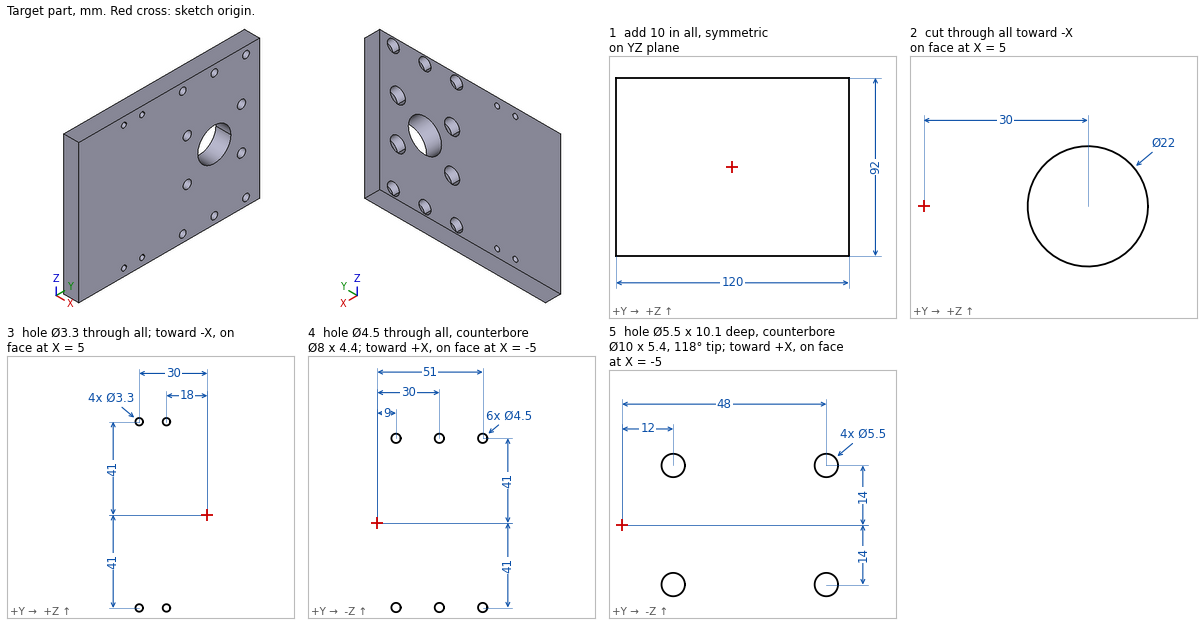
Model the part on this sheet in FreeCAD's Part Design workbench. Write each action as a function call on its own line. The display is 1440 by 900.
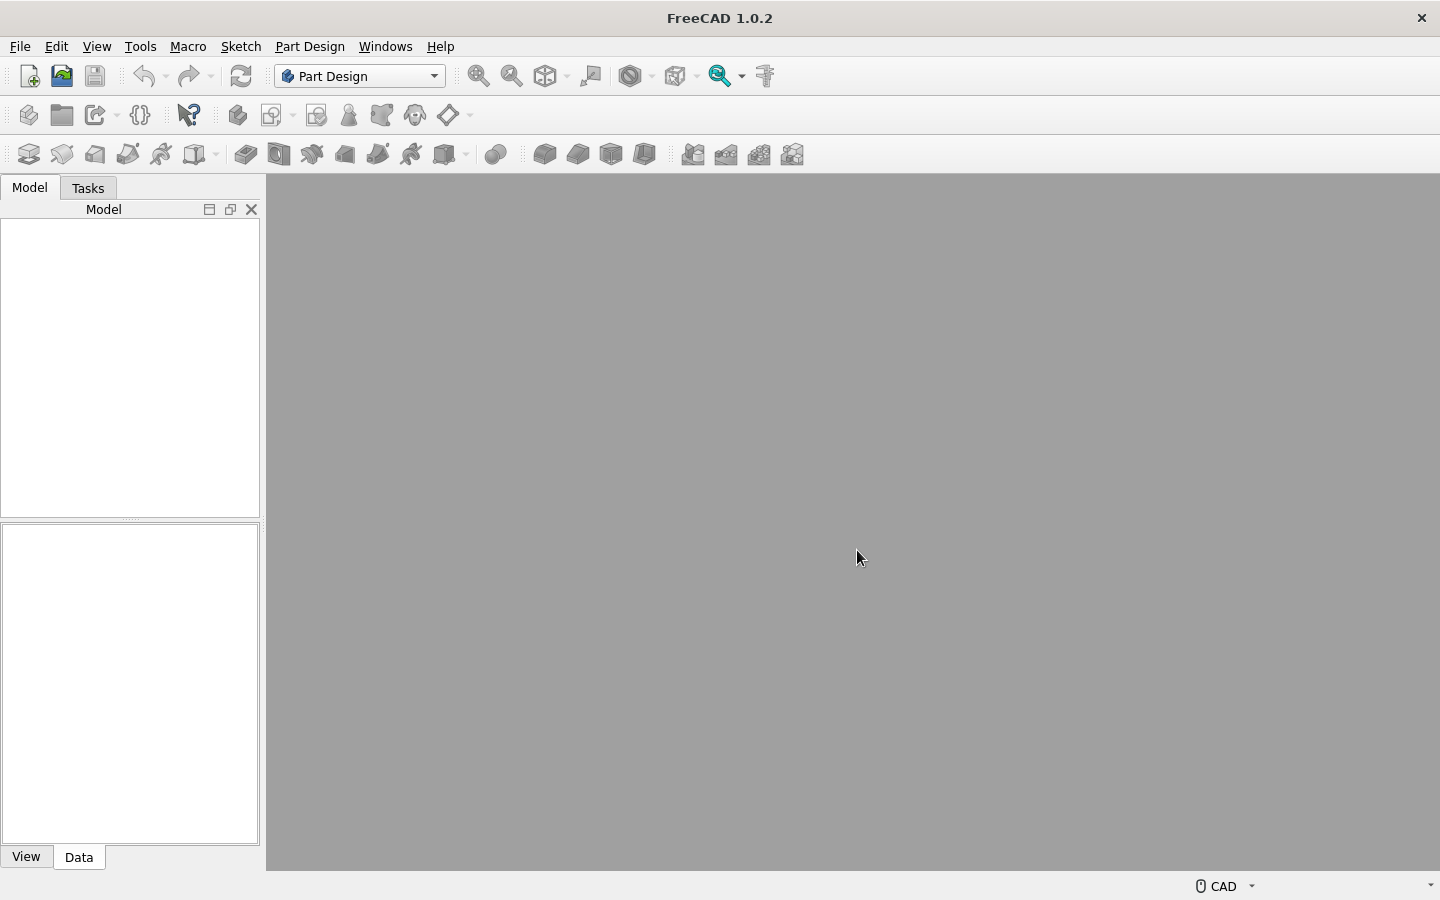
key(ctrl+n)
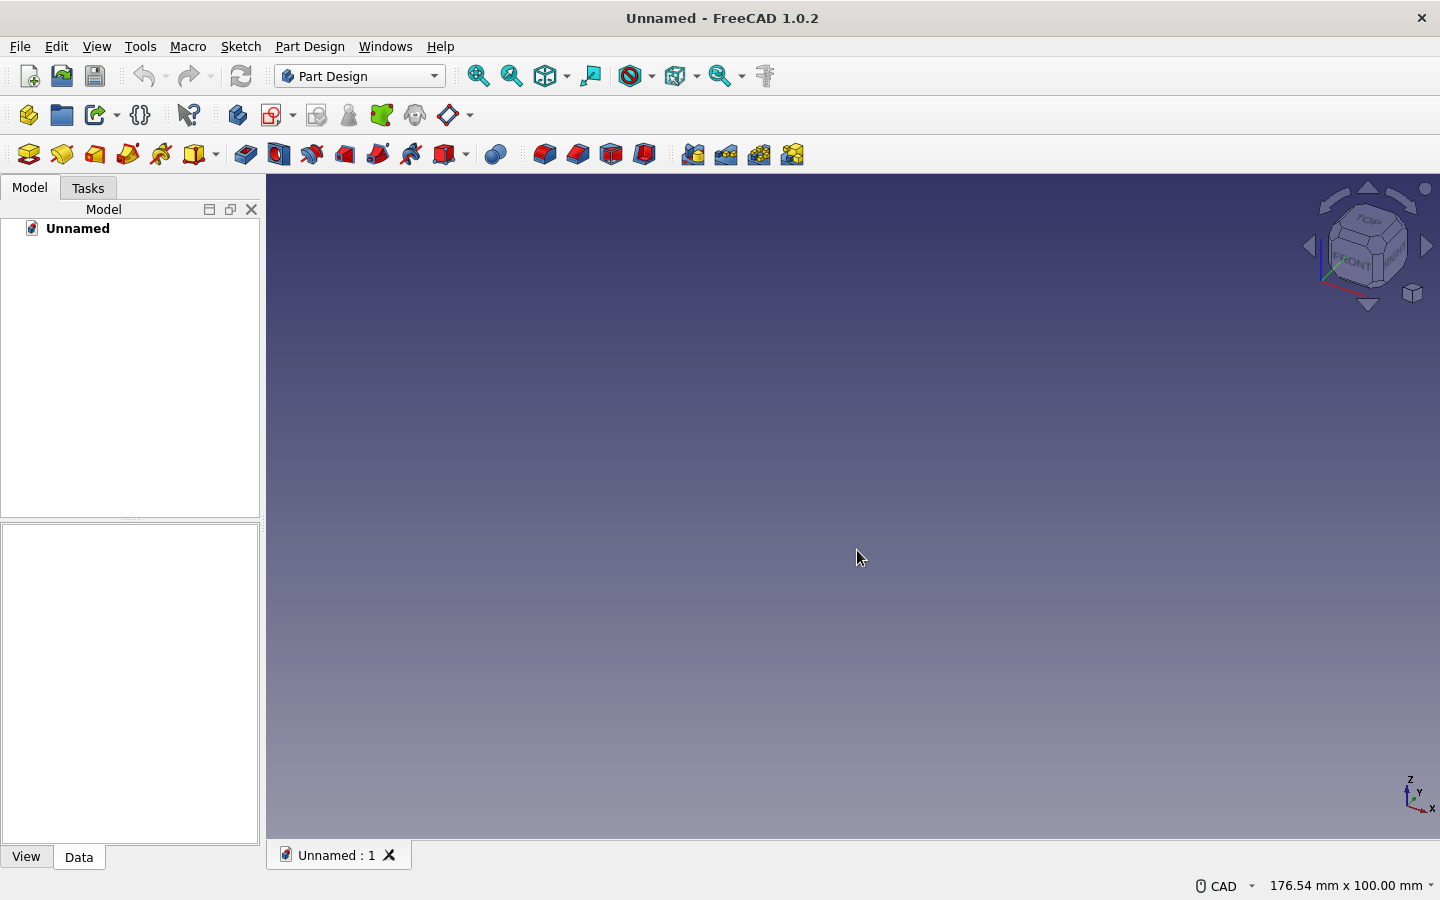
click(270, 116)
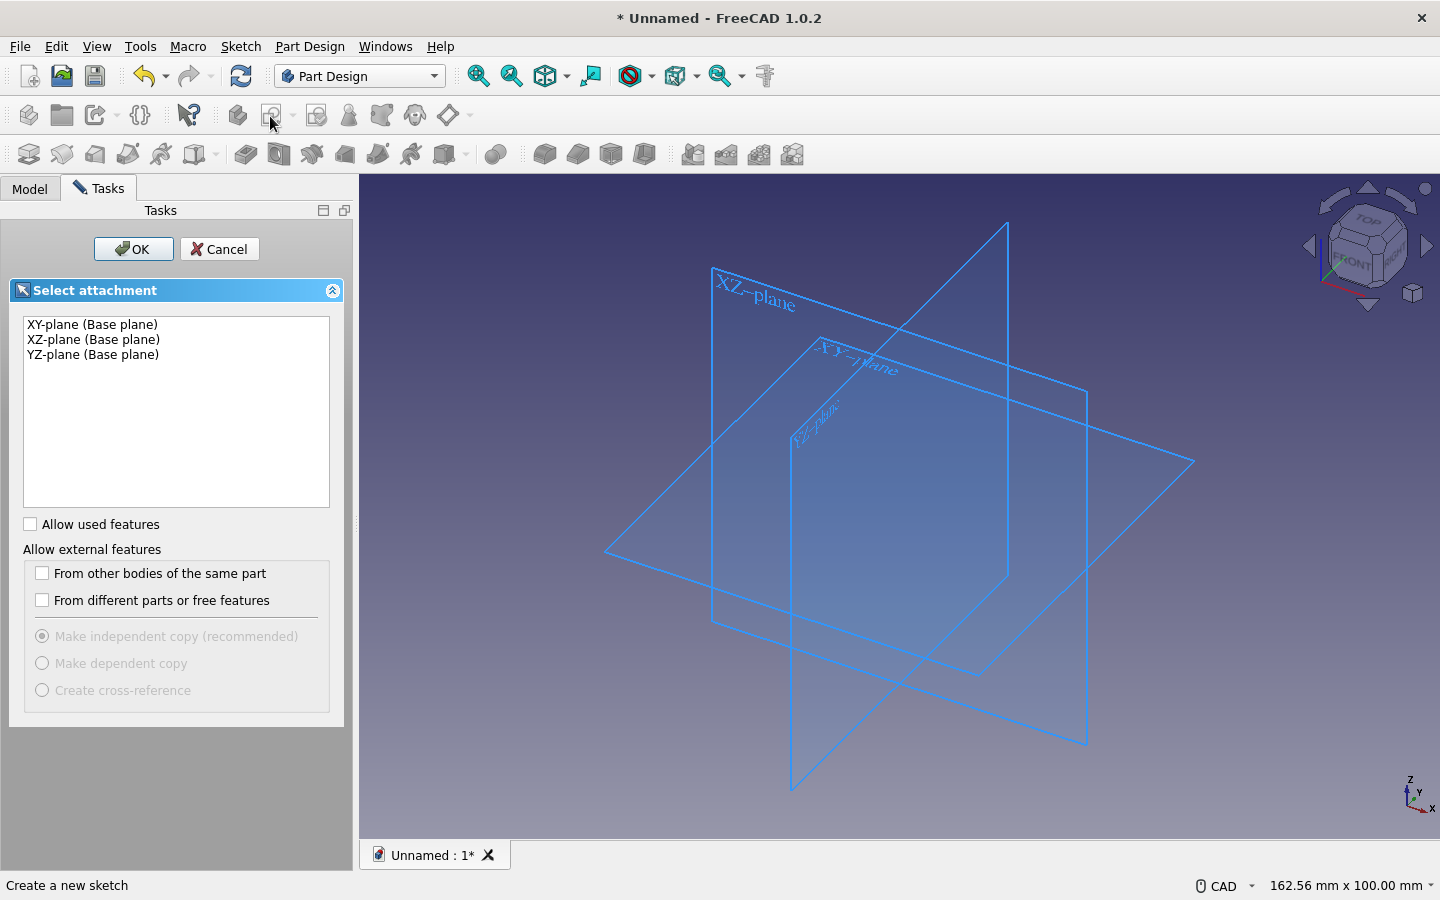
click(84, 354)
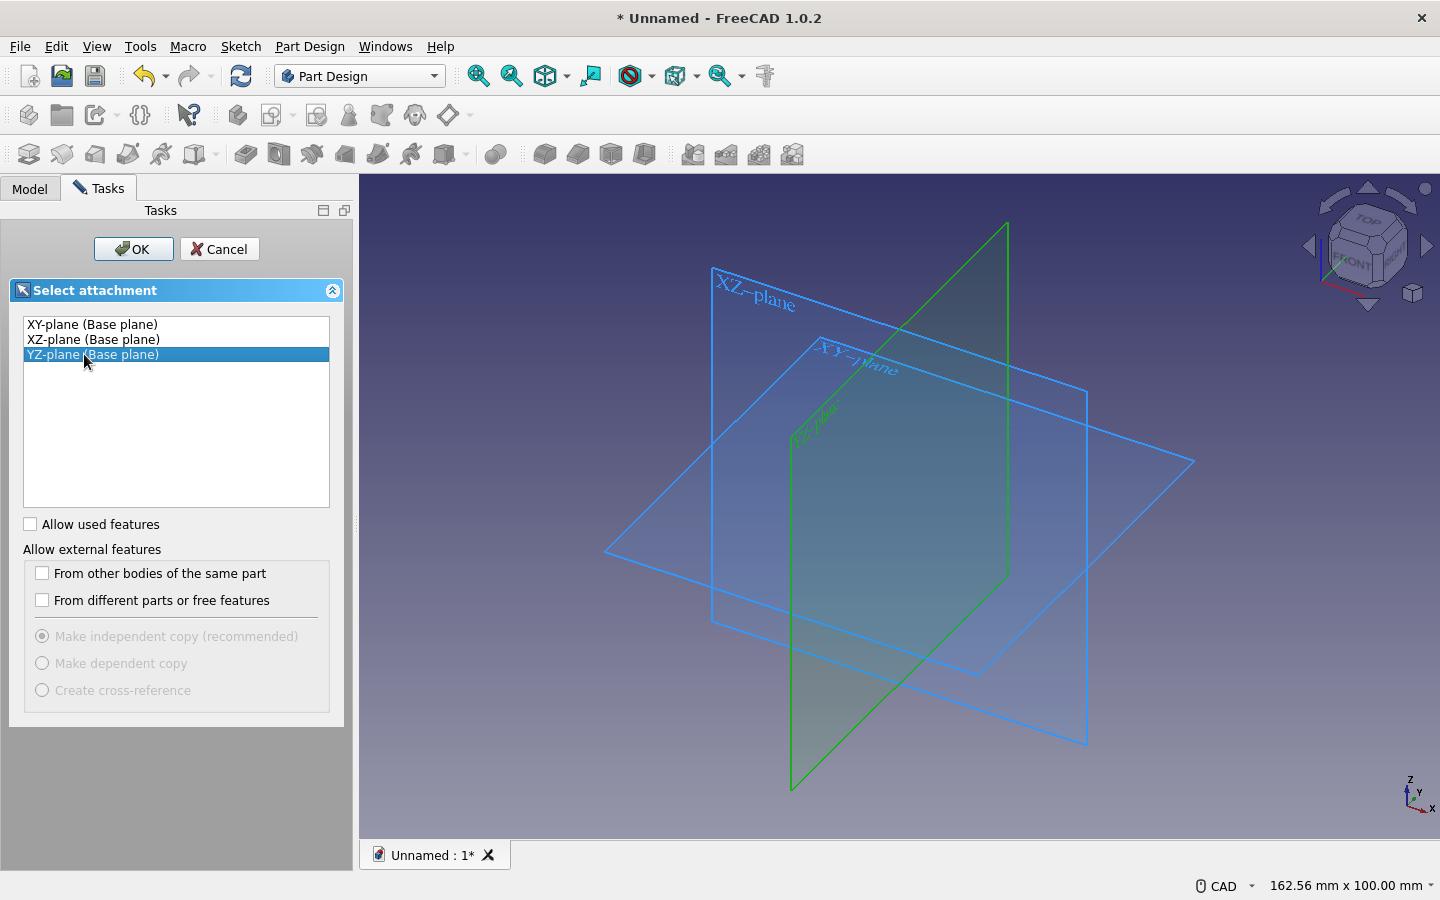
click(134, 249)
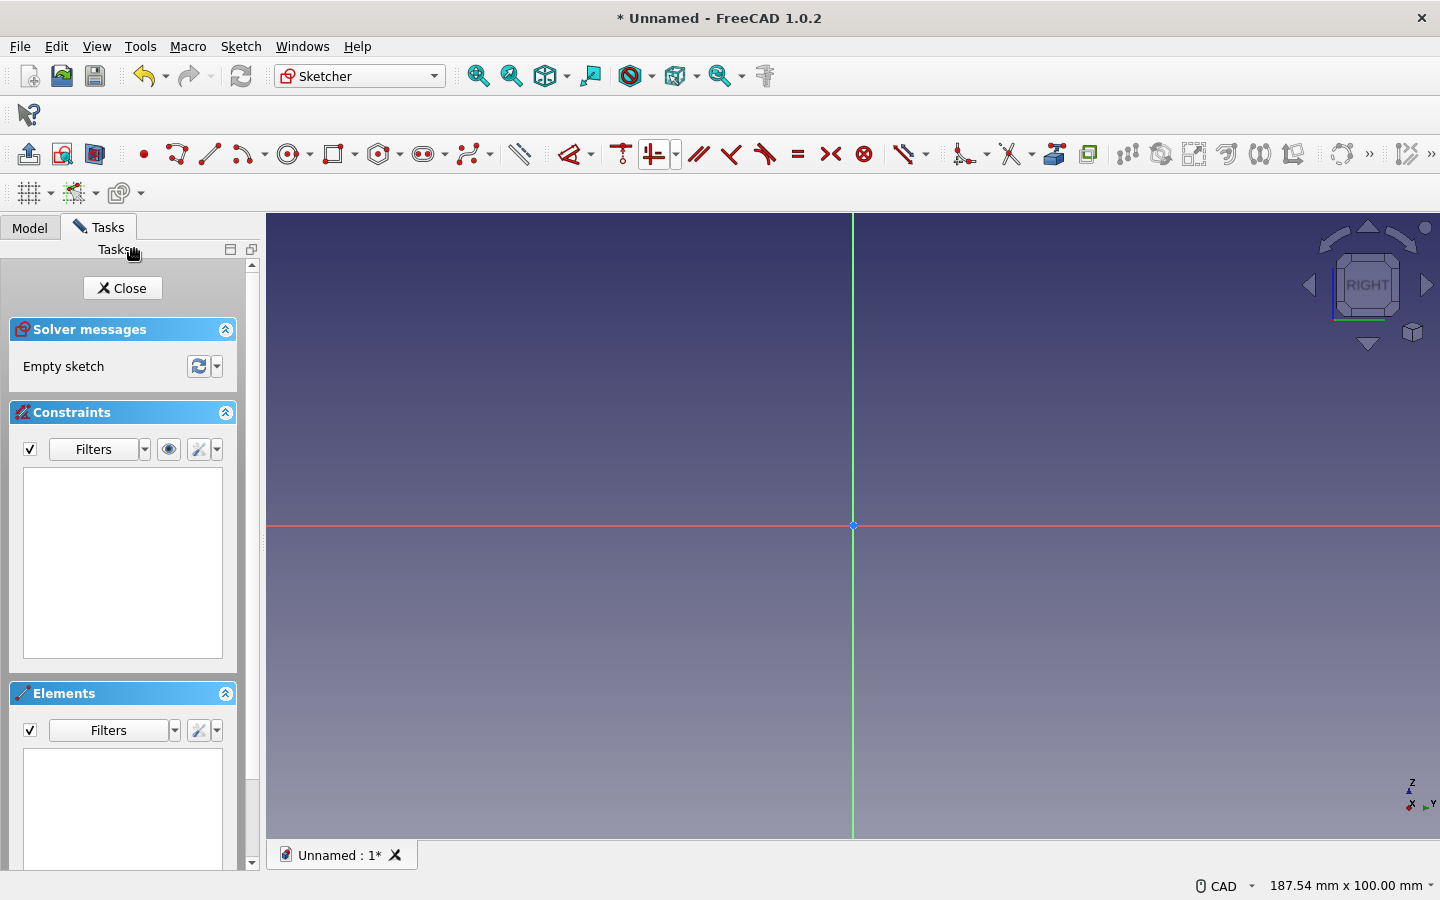
scroll(645, 526, down, 2)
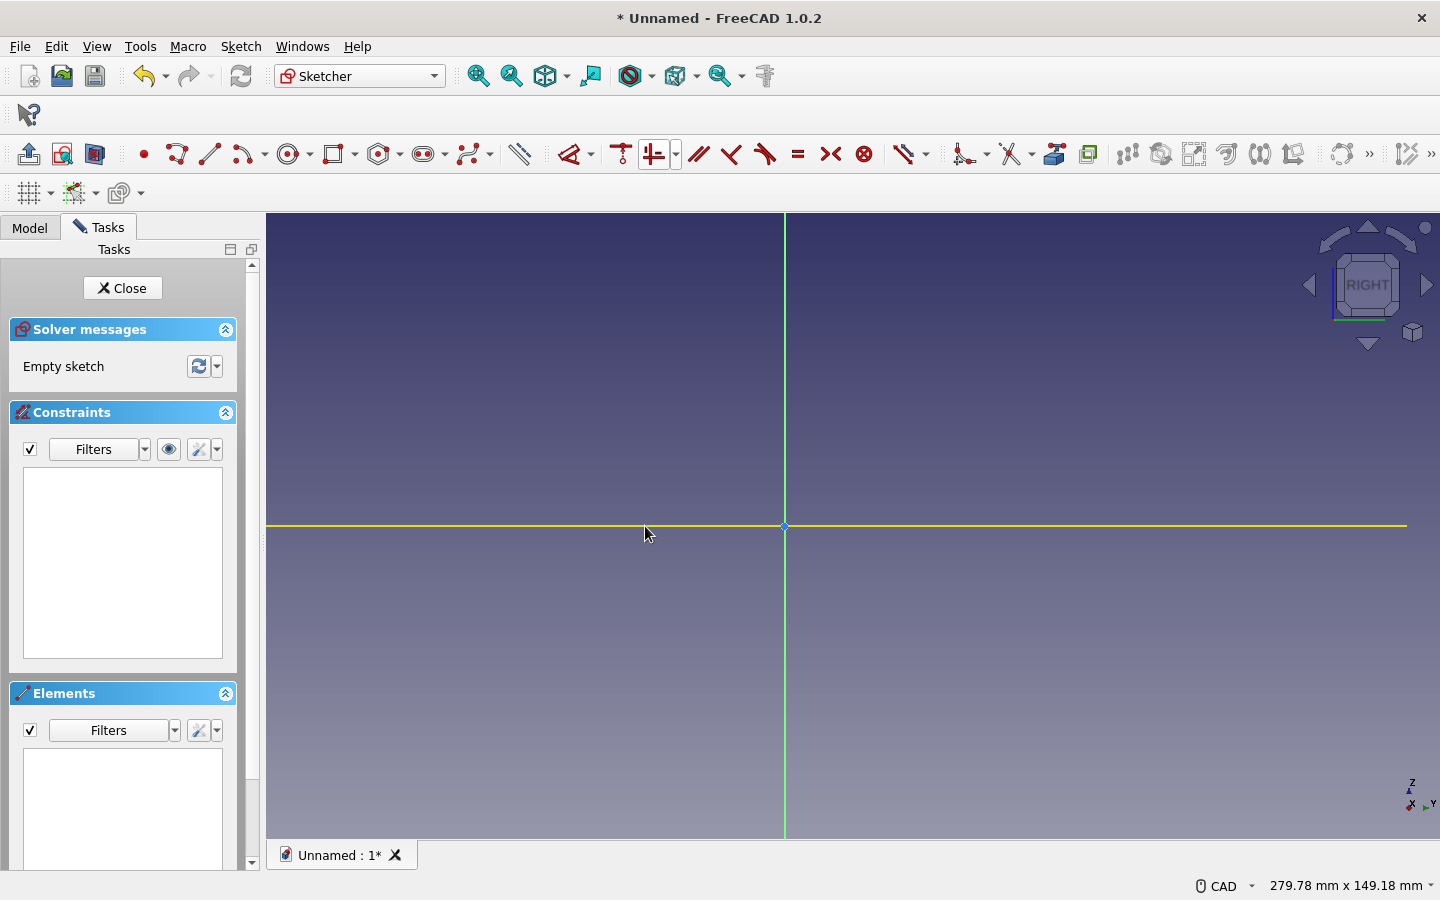
key(g)
key(v)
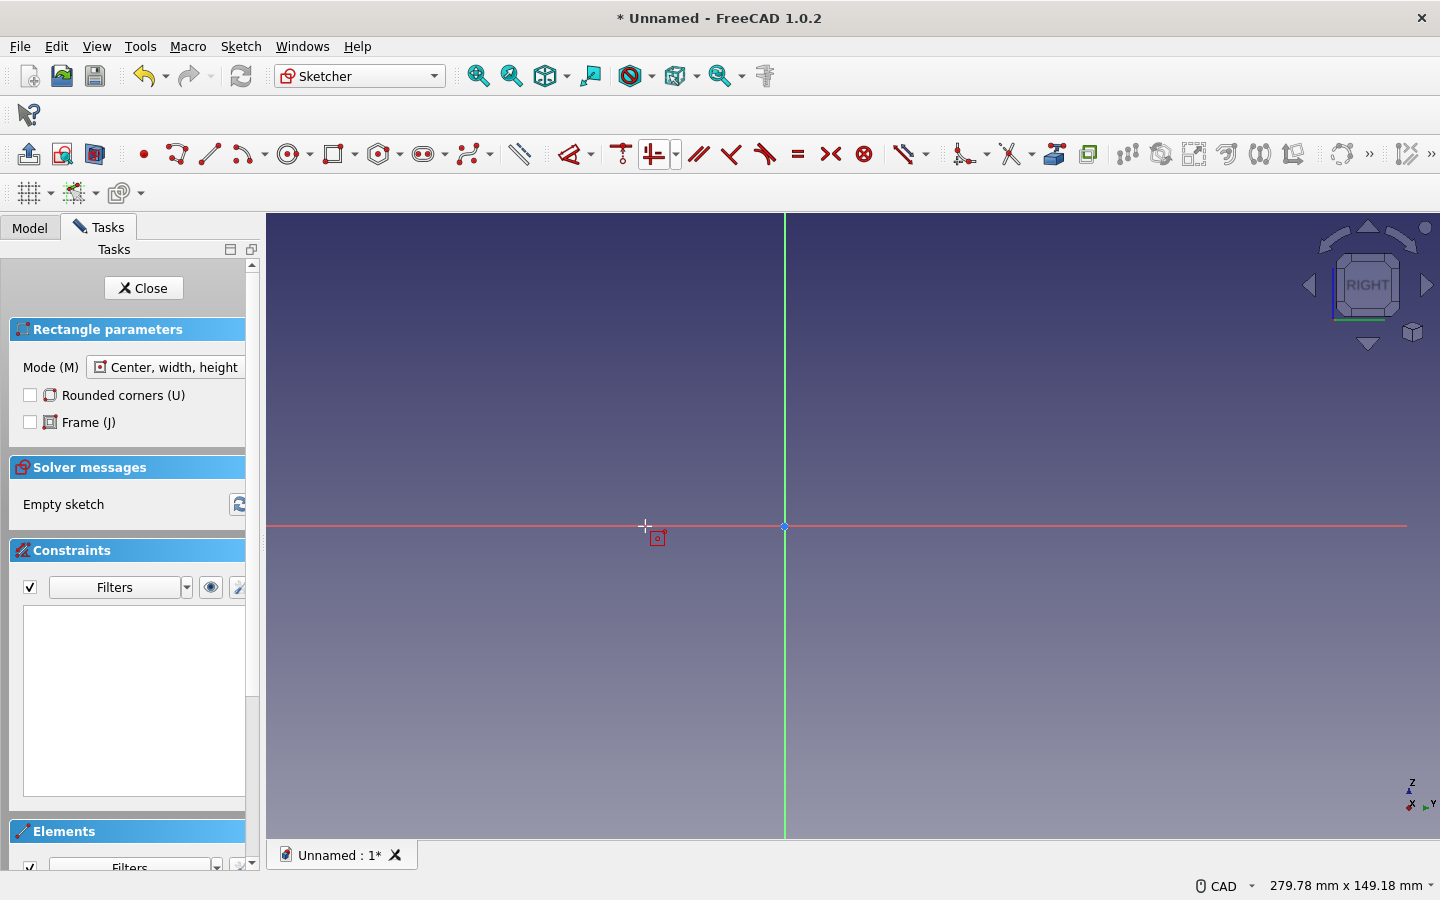
click(785, 526)
click(1036, 333)
key(Escape)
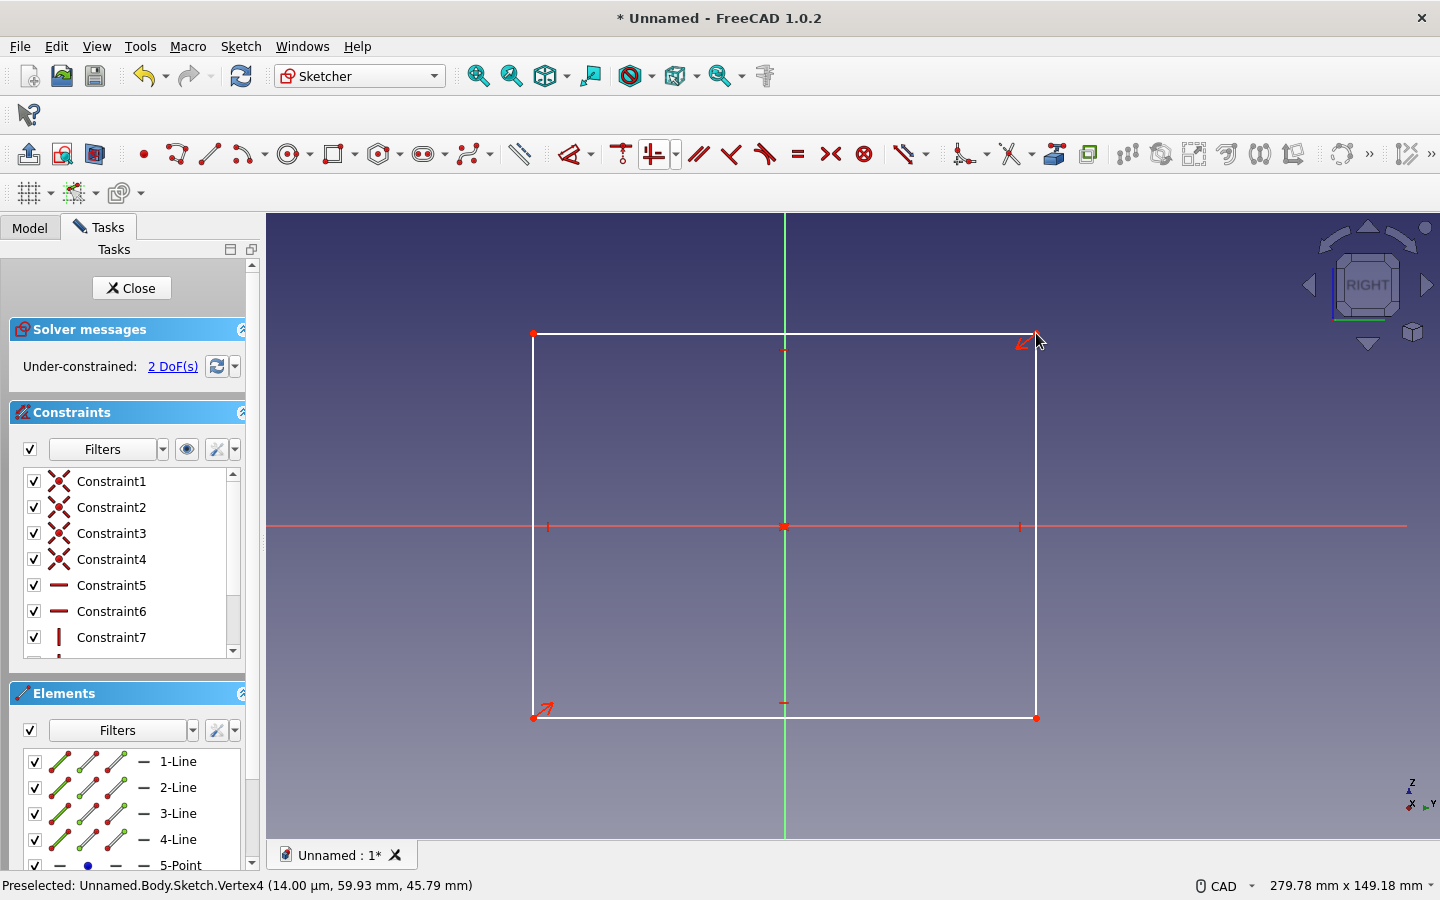
click(568, 154)